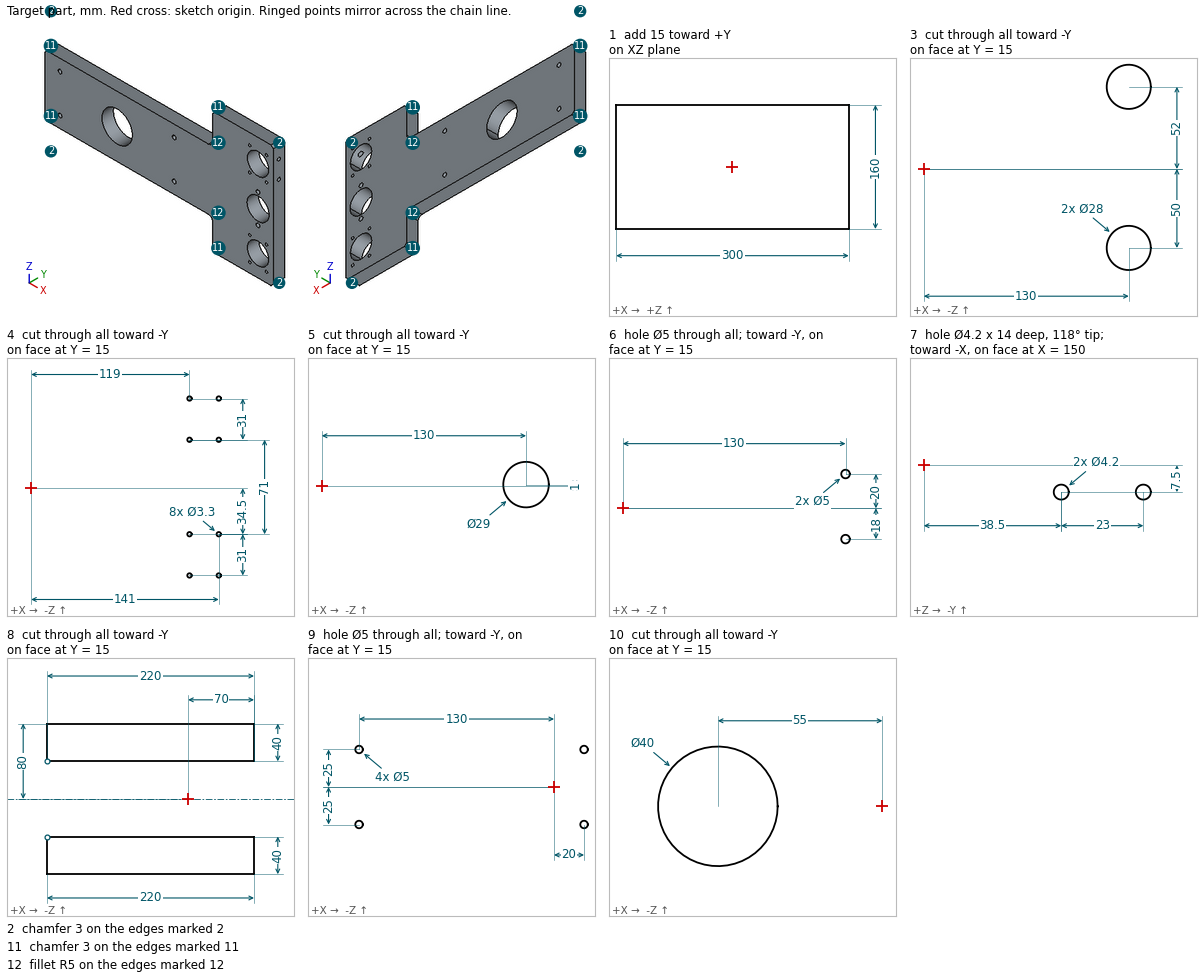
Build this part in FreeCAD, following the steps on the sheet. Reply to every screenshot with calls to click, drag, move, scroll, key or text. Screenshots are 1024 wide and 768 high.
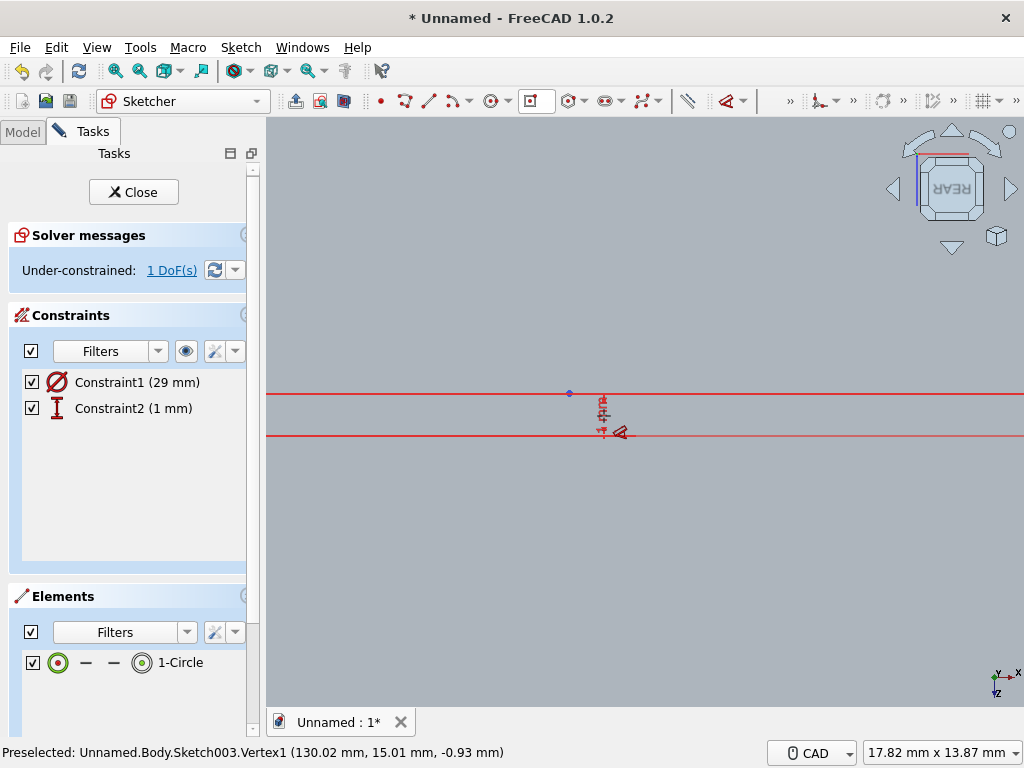
click(570, 394)
click(432, 470)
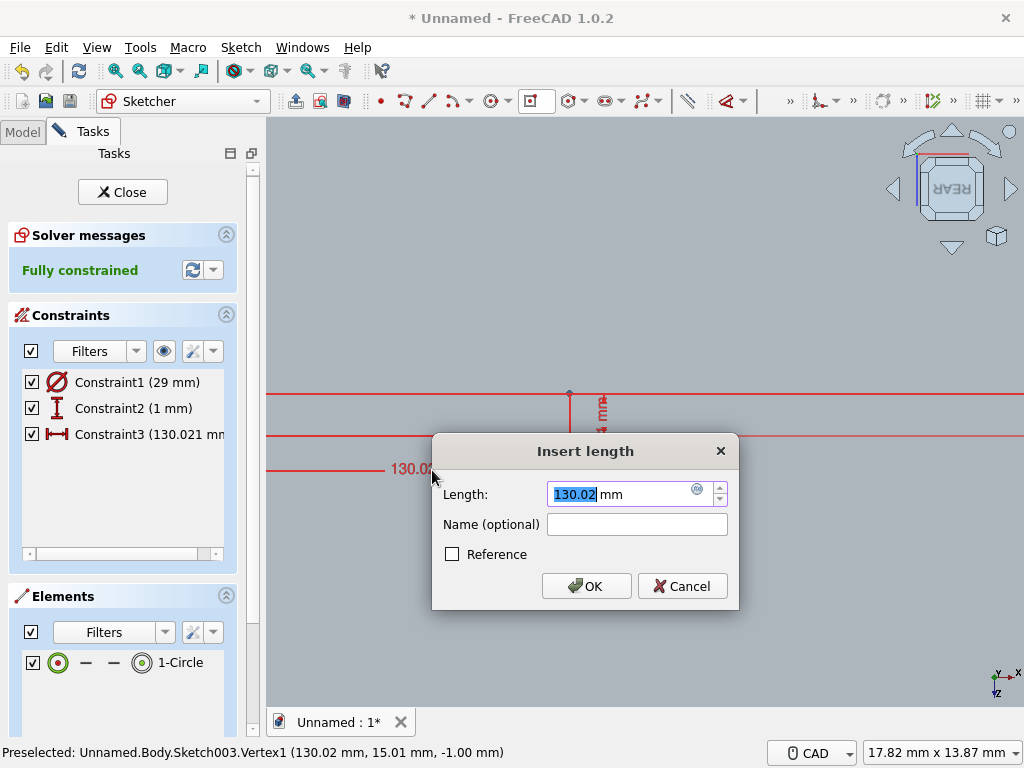
text(130)
key(Return)
key(Escape)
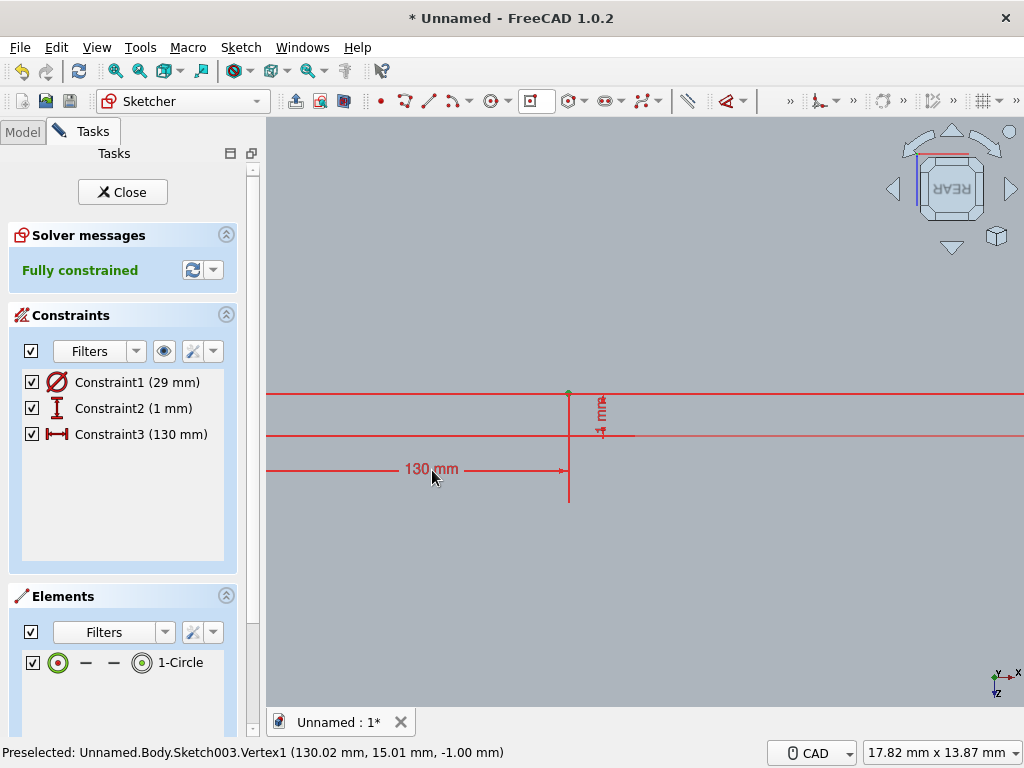
click(123, 192)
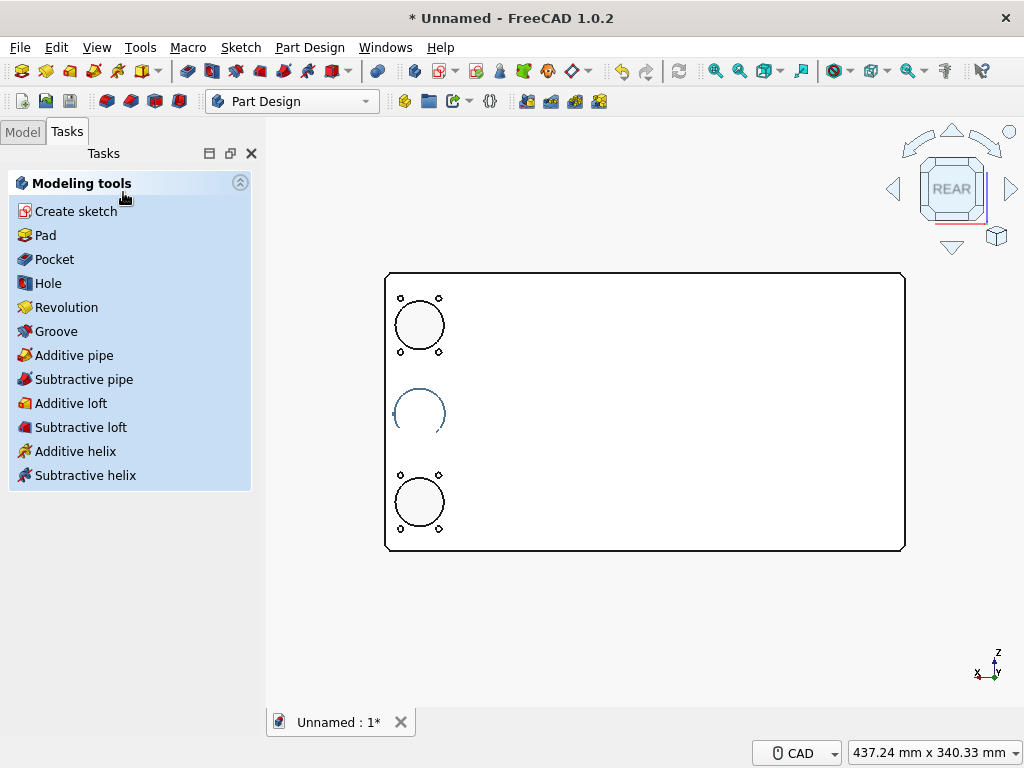
click(188, 72)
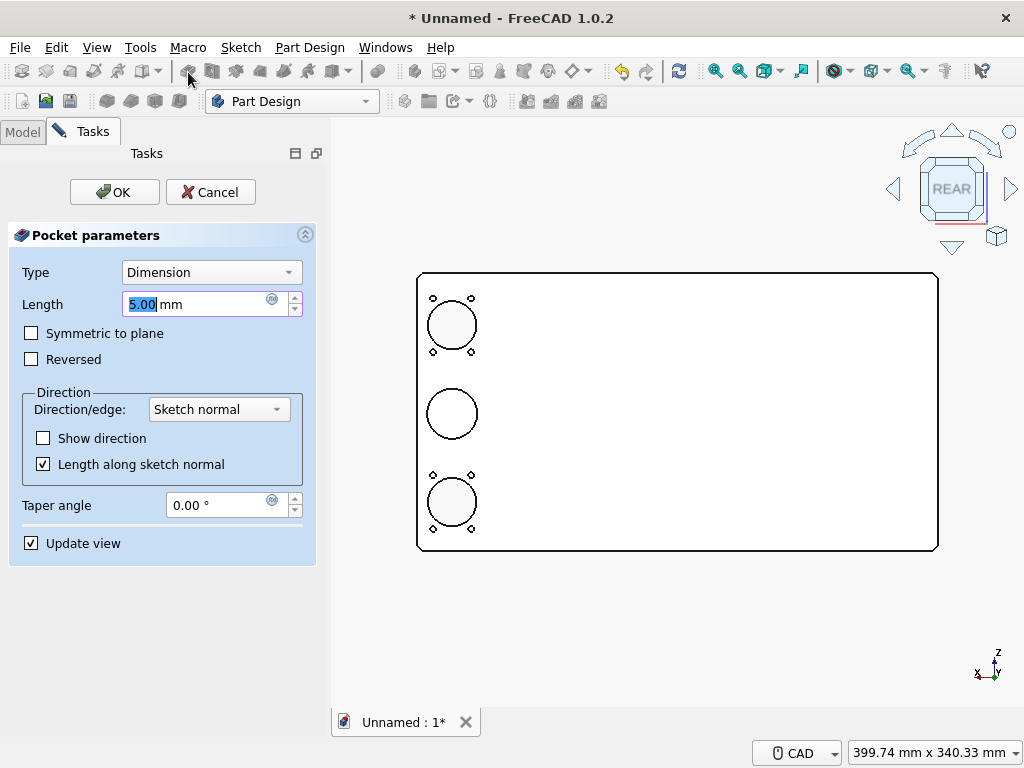
click(212, 272)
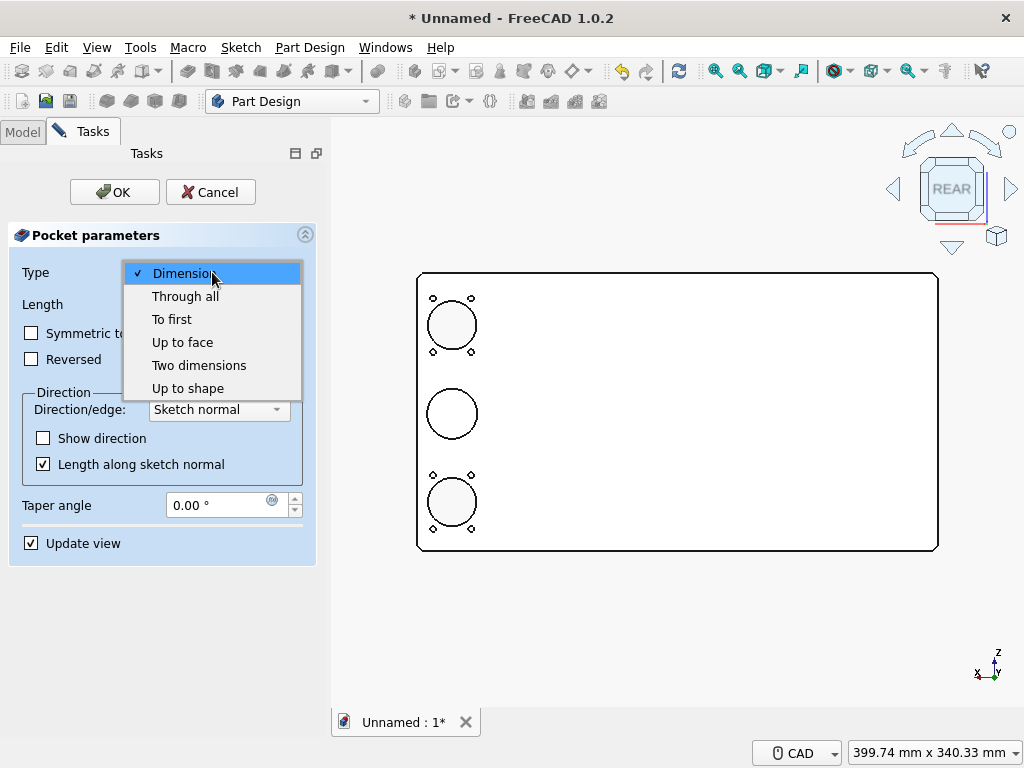
click(212, 296)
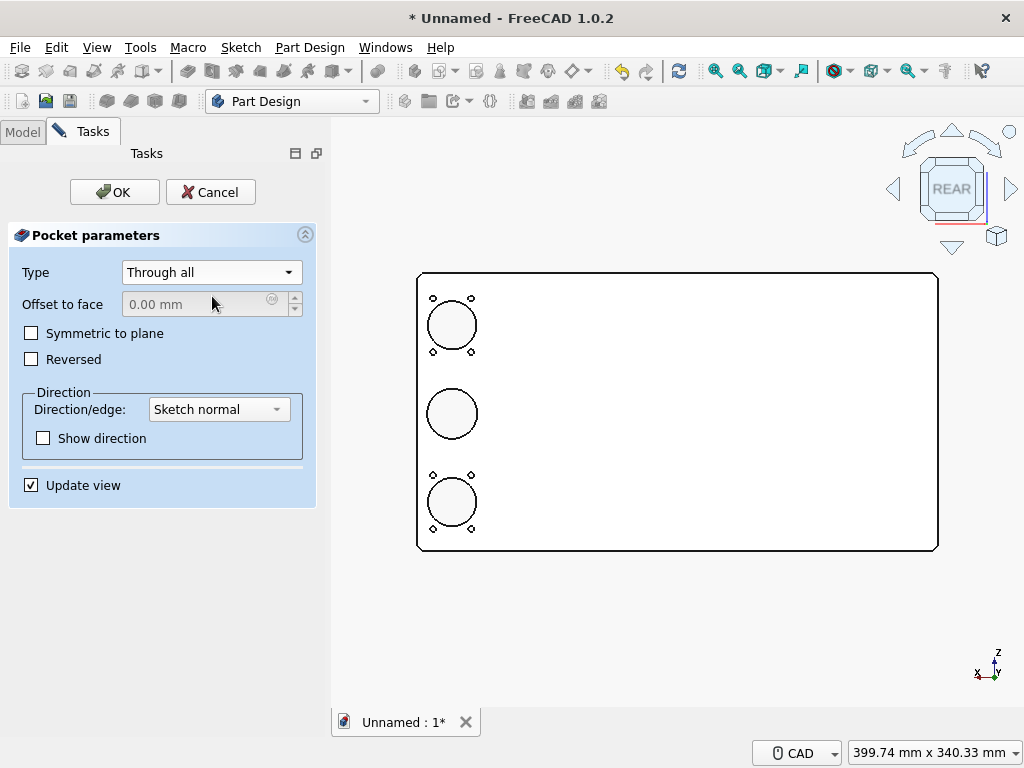
click(115, 192)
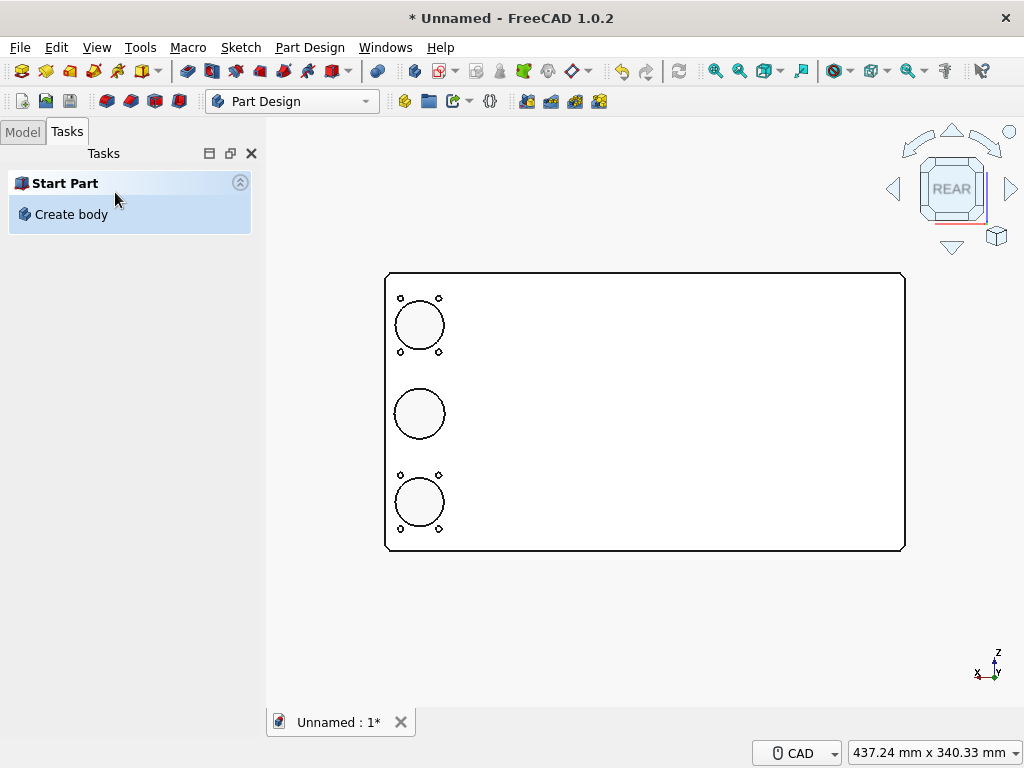
click(645, 411)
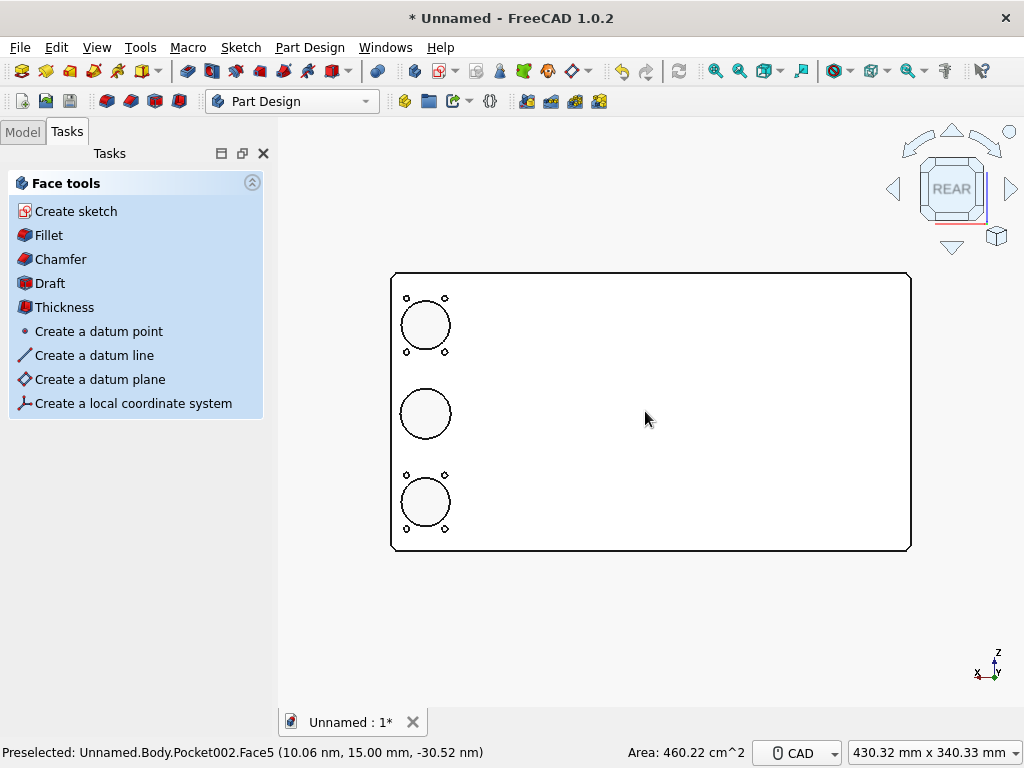
click(440, 72)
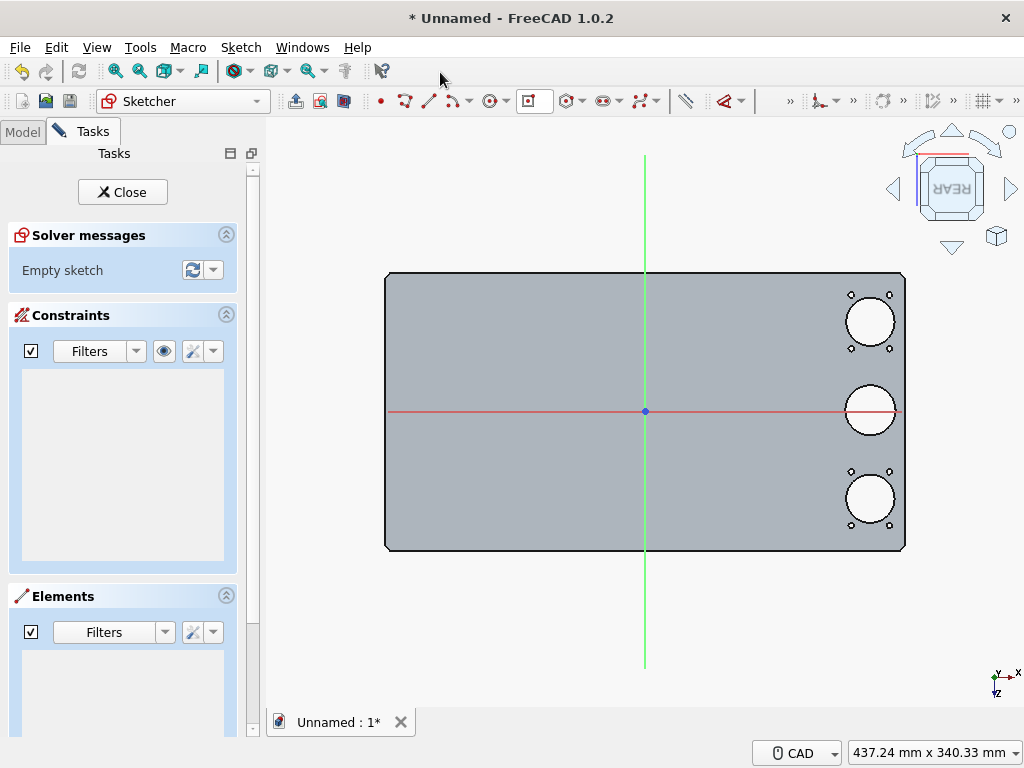
scroll(576, 412, down, 5)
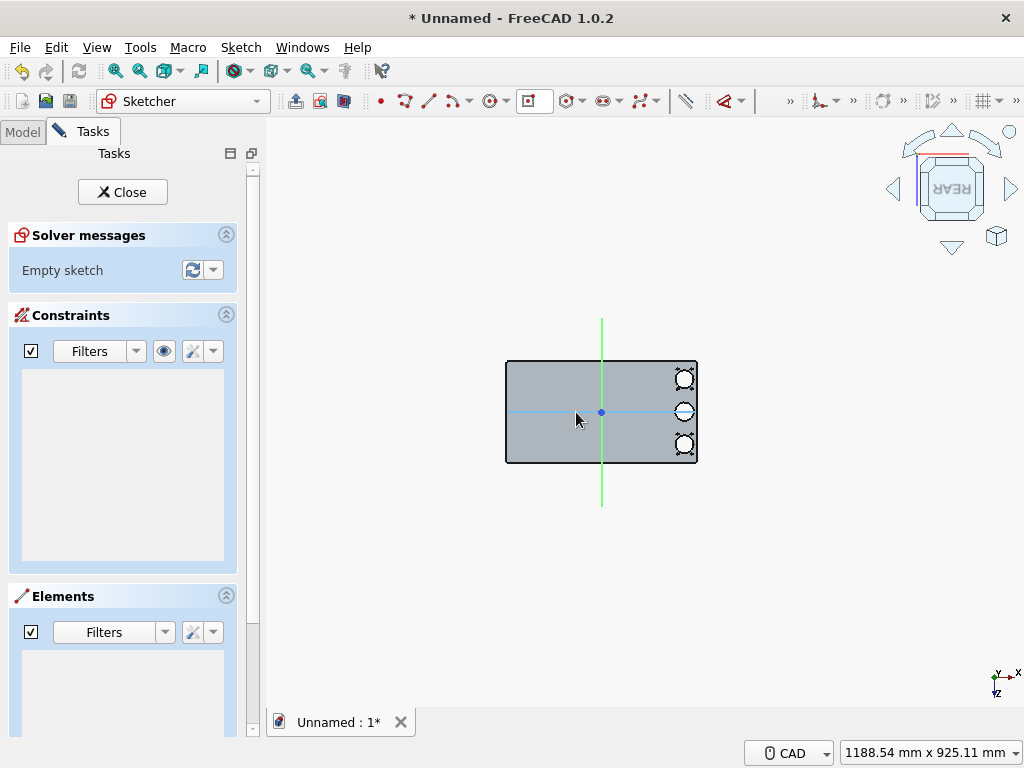
scroll(693, 412, up, 13)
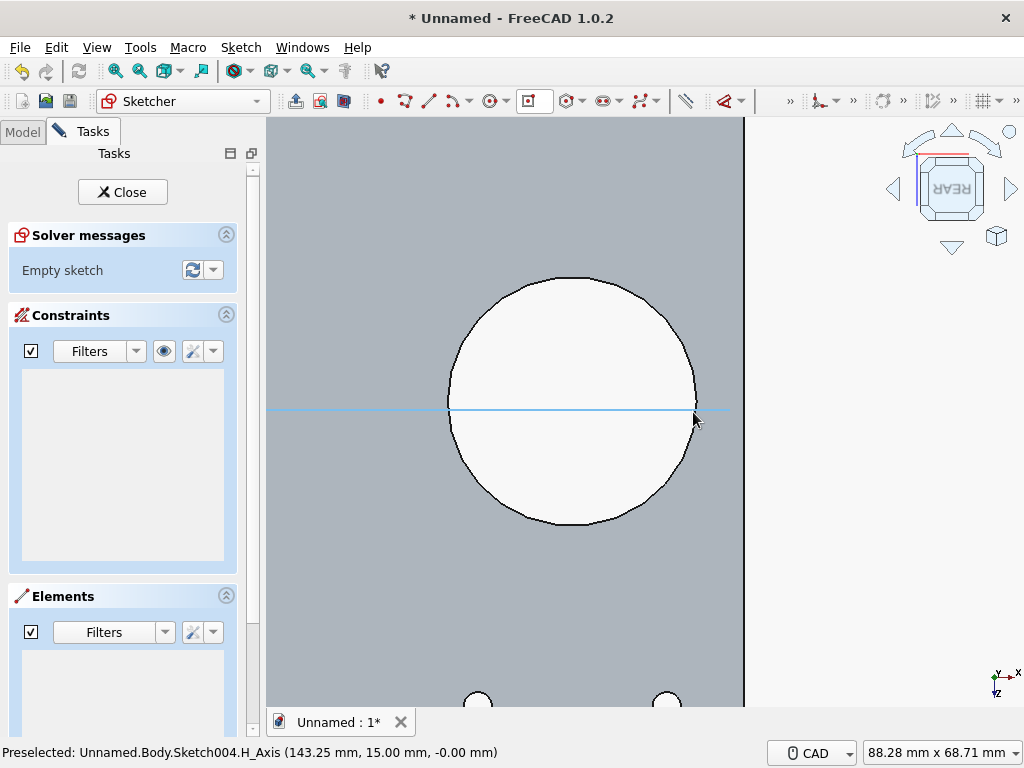
click(490, 102)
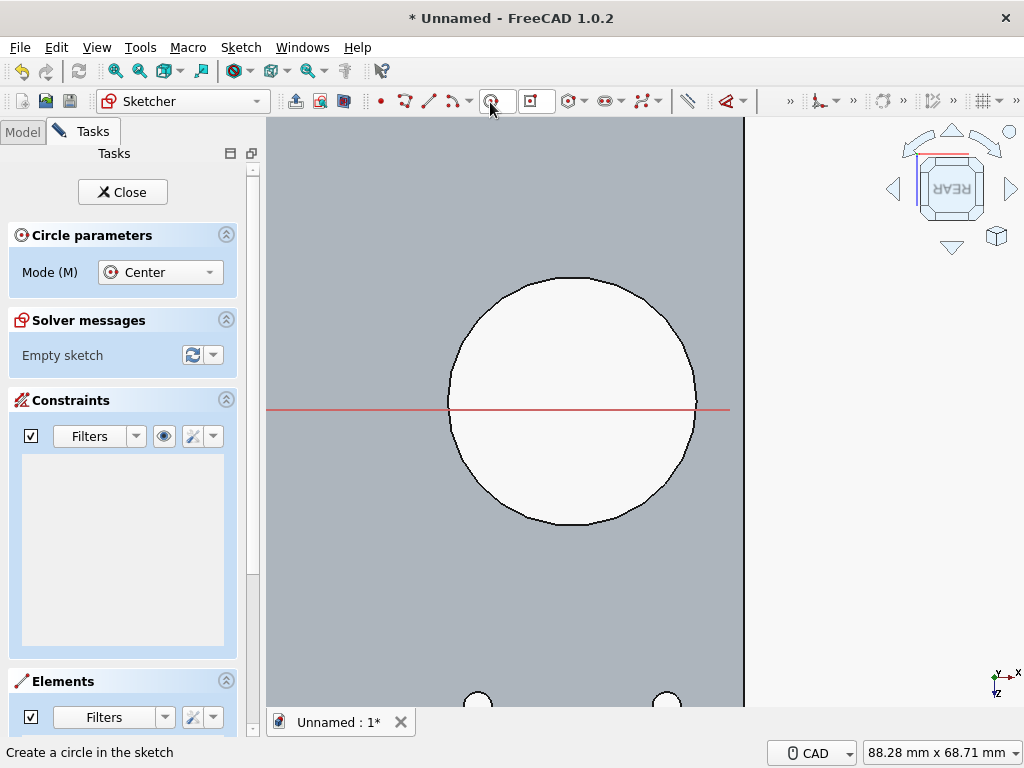
click(572, 238)
move(587, 223)